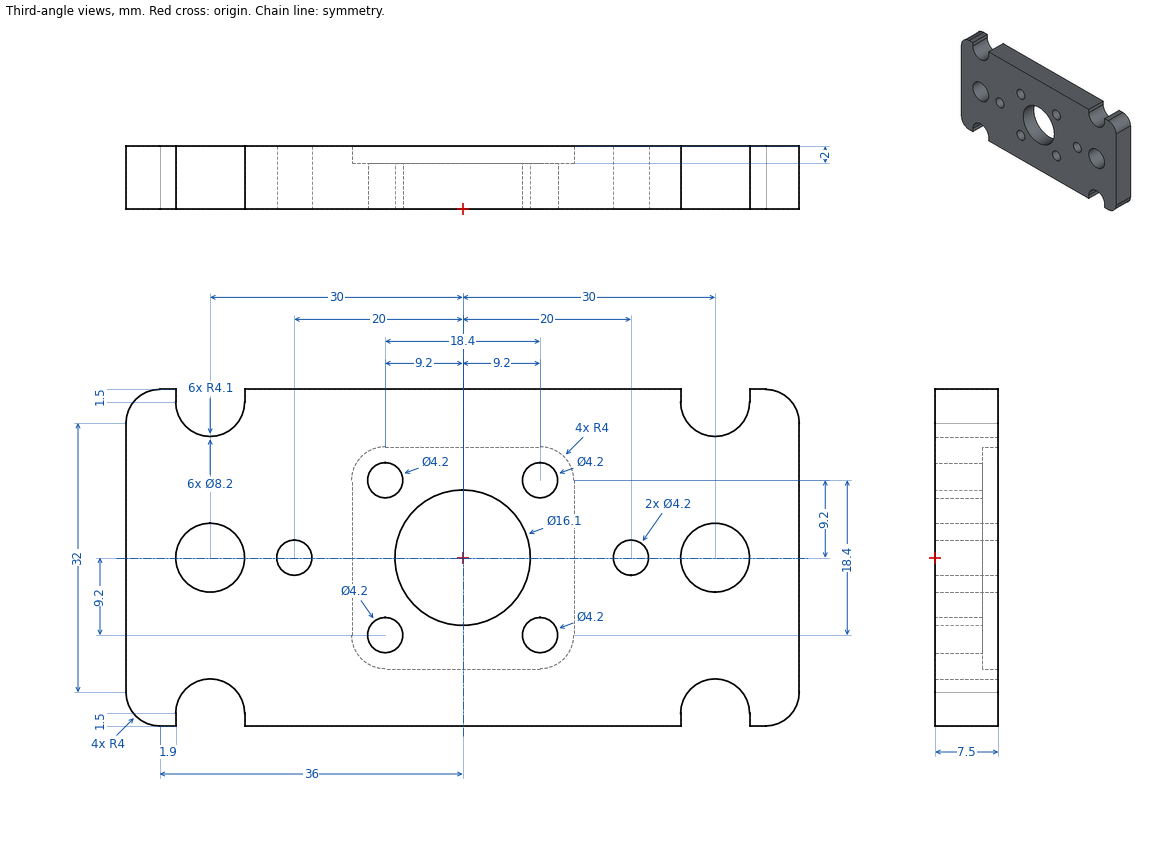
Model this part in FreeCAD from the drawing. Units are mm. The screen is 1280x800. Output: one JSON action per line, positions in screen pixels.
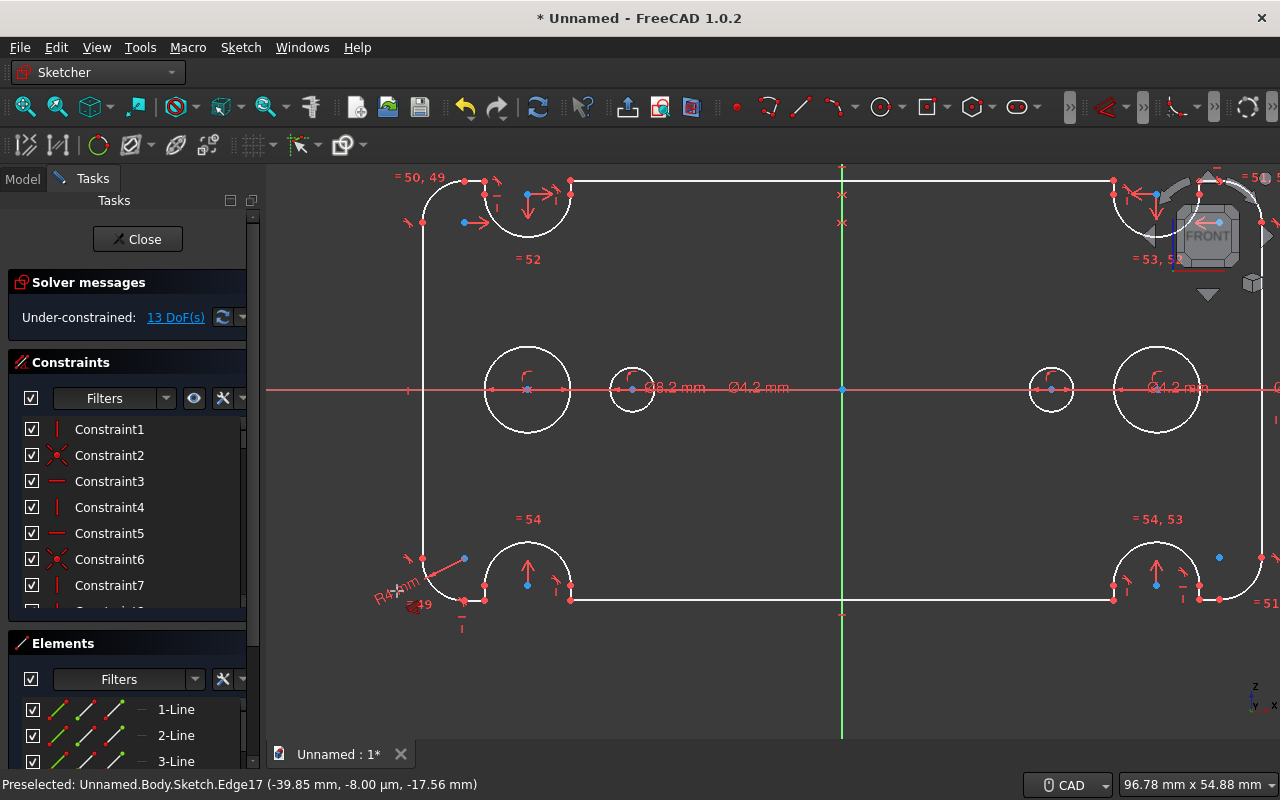
{"action": "left_click", "coordinate": [503, 229]}
{"action": "left_click", "coordinate": [484, 255]}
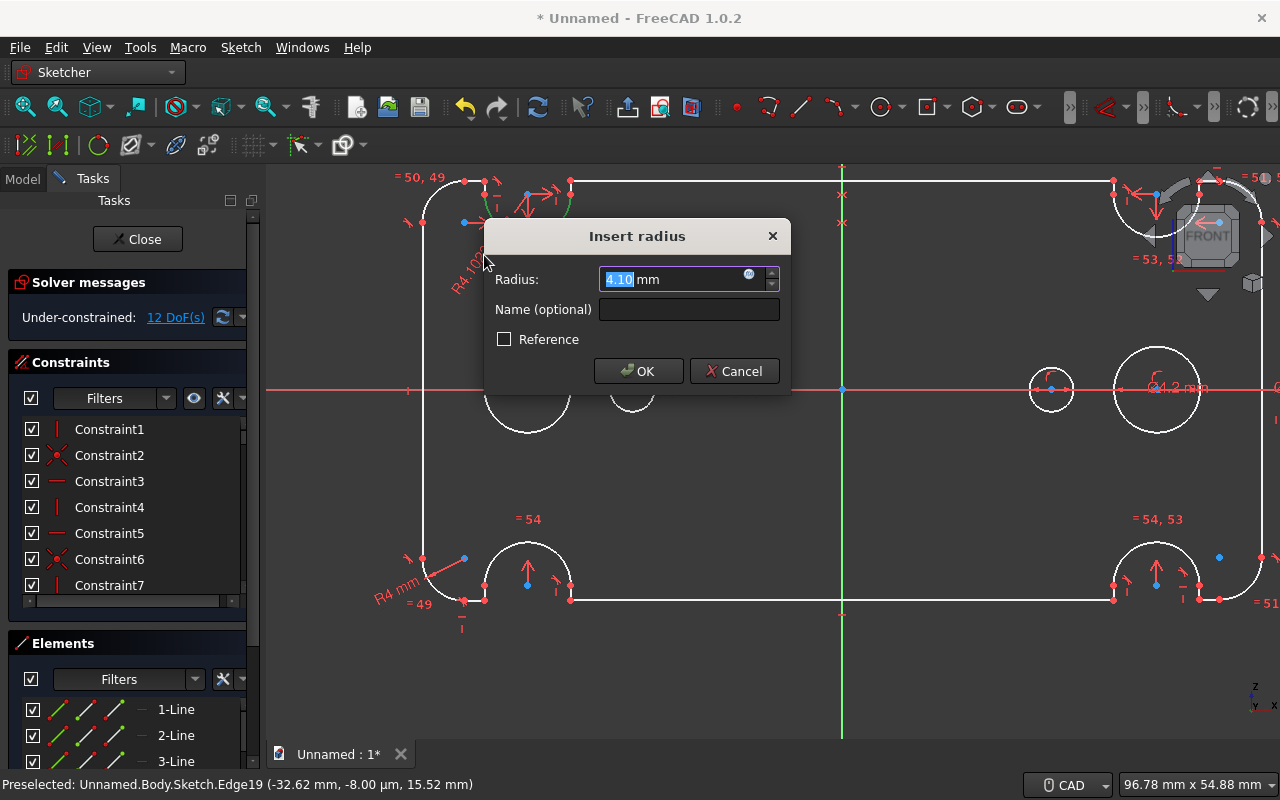
{"action": "type", "text": "4.1"}
{"action": "key", "text": "Return"}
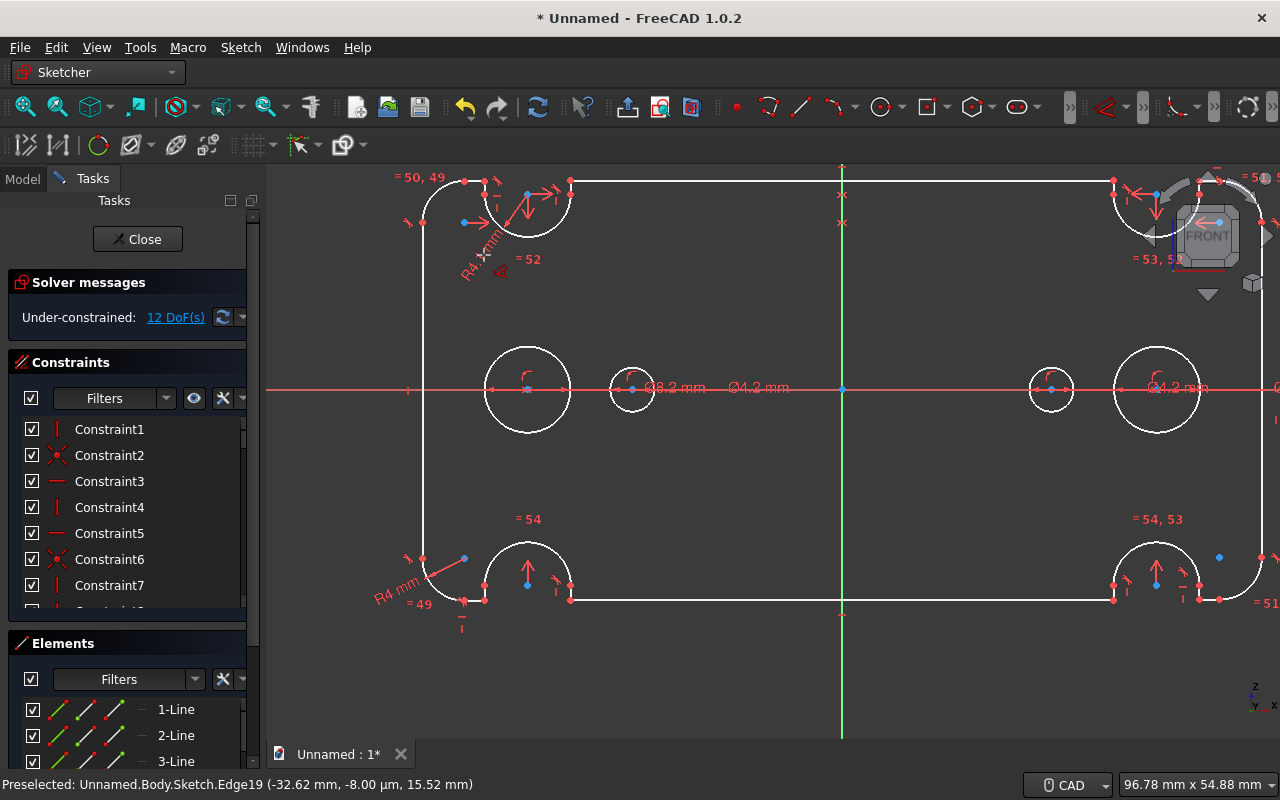
{"action": "left_click", "coordinate": [423, 458]}
{"action": "left_click", "coordinate": [389, 314]}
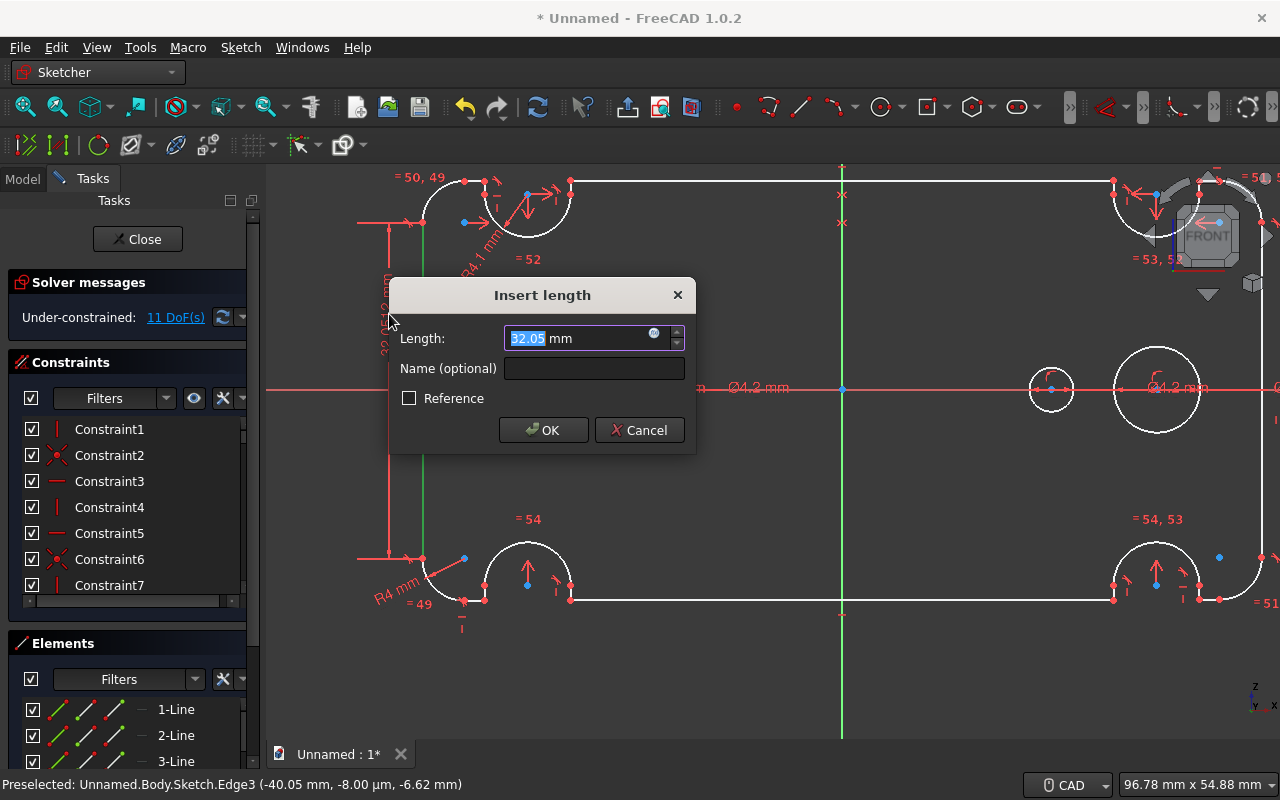
{"action": "type", "text": "32"}
{"action": "key", "text": "Return"}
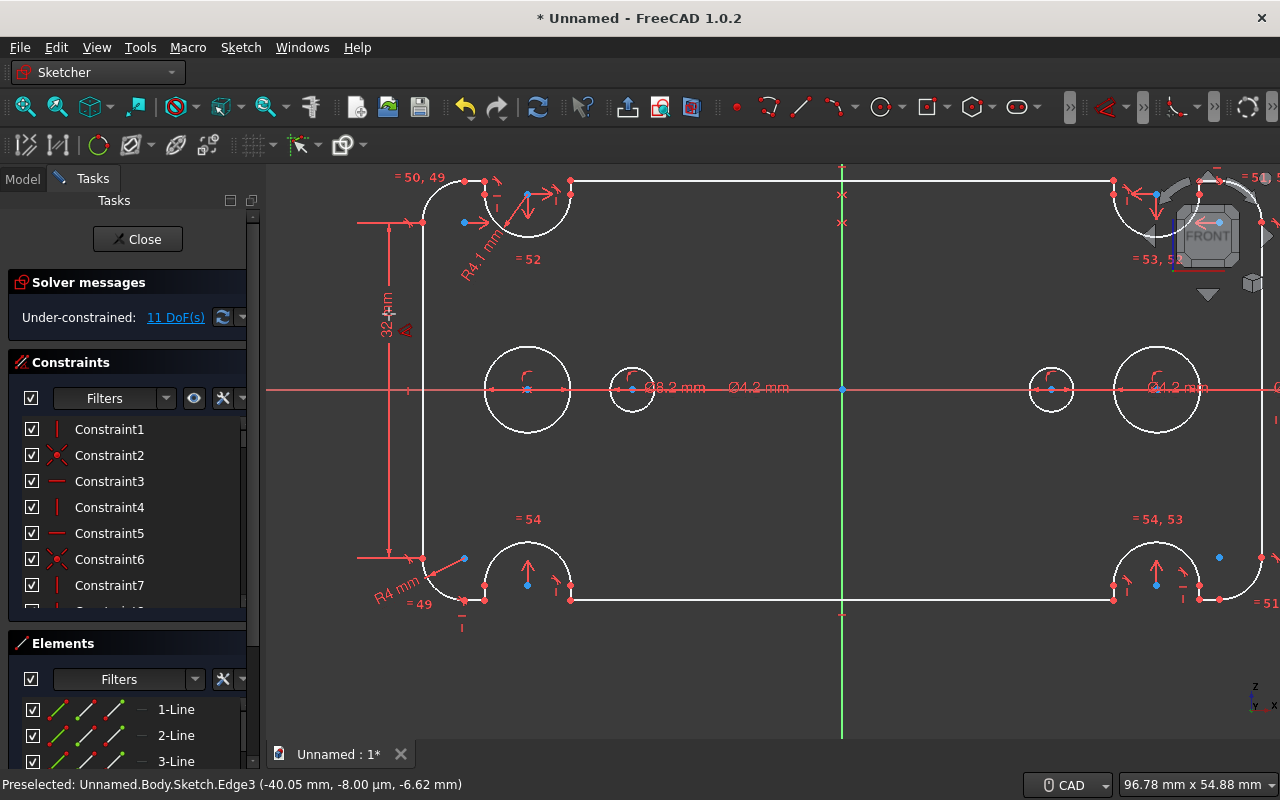
{"action": "scroll", "coordinate": [425, 577], "scroll_direction": "down", "scroll_amount": 2}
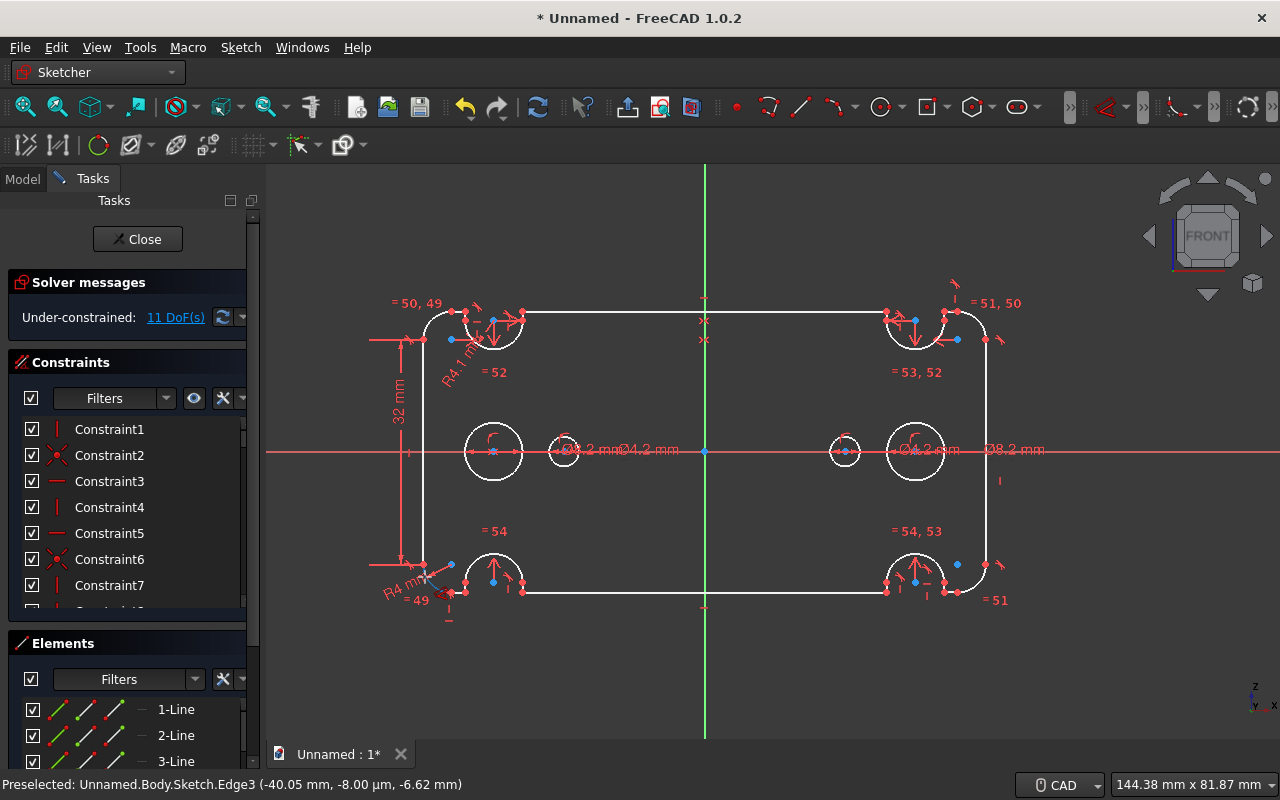
{"action": "left_click", "coordinate": [986, 407]}
{"action": "left_click", "coordinate": [1020, 400]}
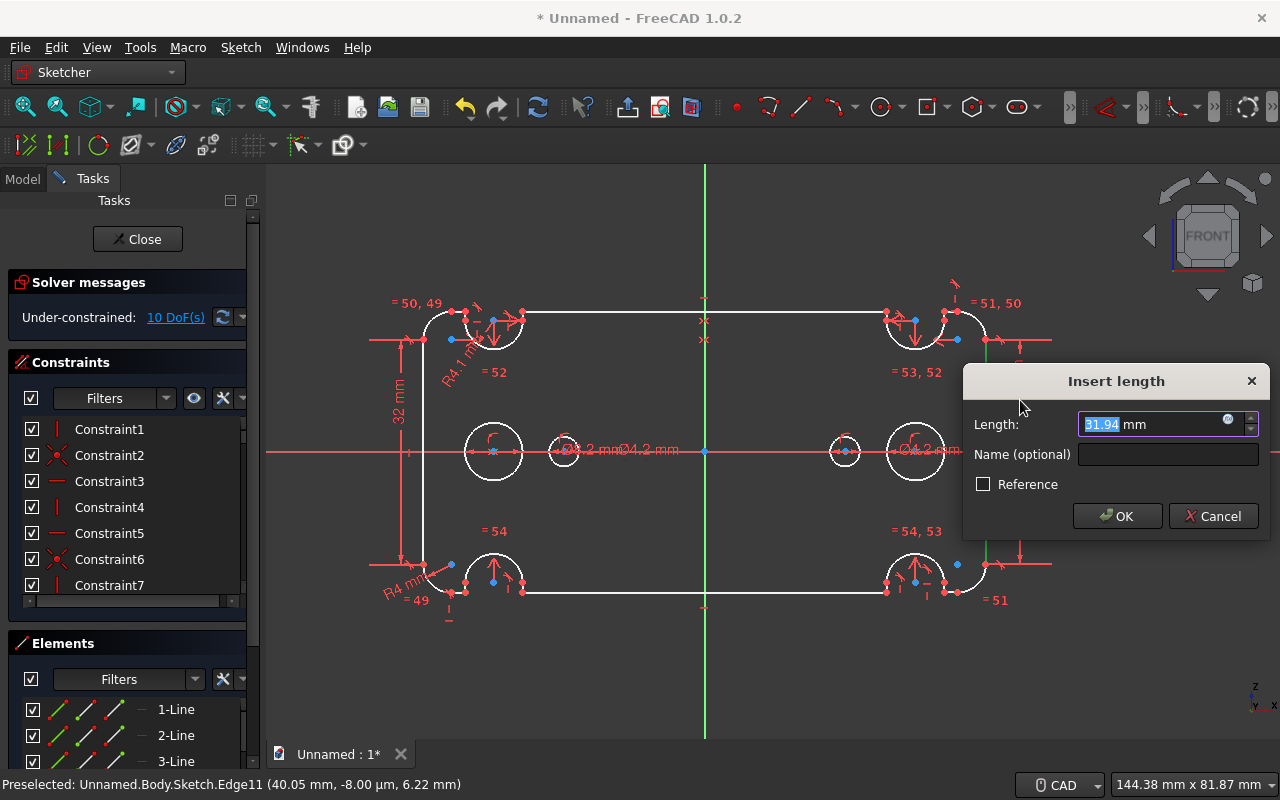
{"action": "type", "text": "32"}
{"action": "key", "text": "Return"}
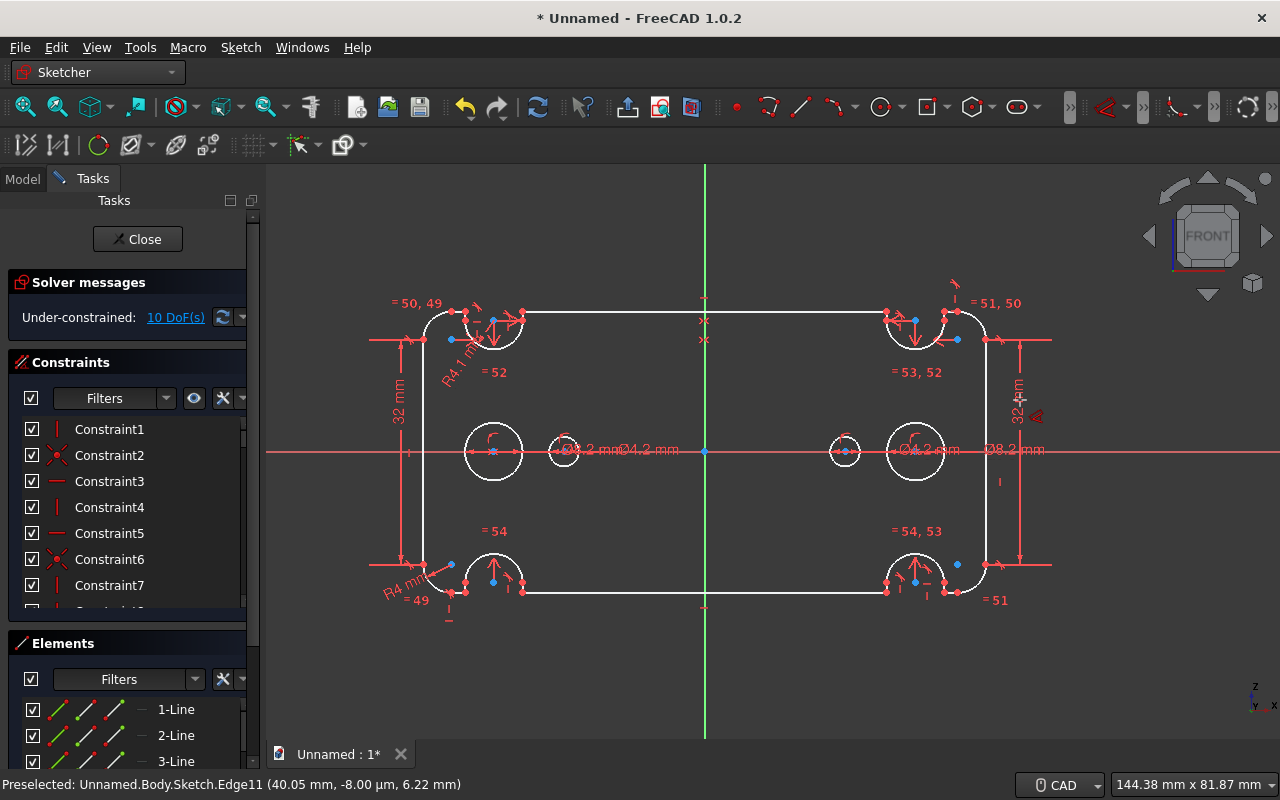
{"action": "left_click", "coordinate": [916, 452]}
{"action": "left_click", "coordinate": [810, 486]}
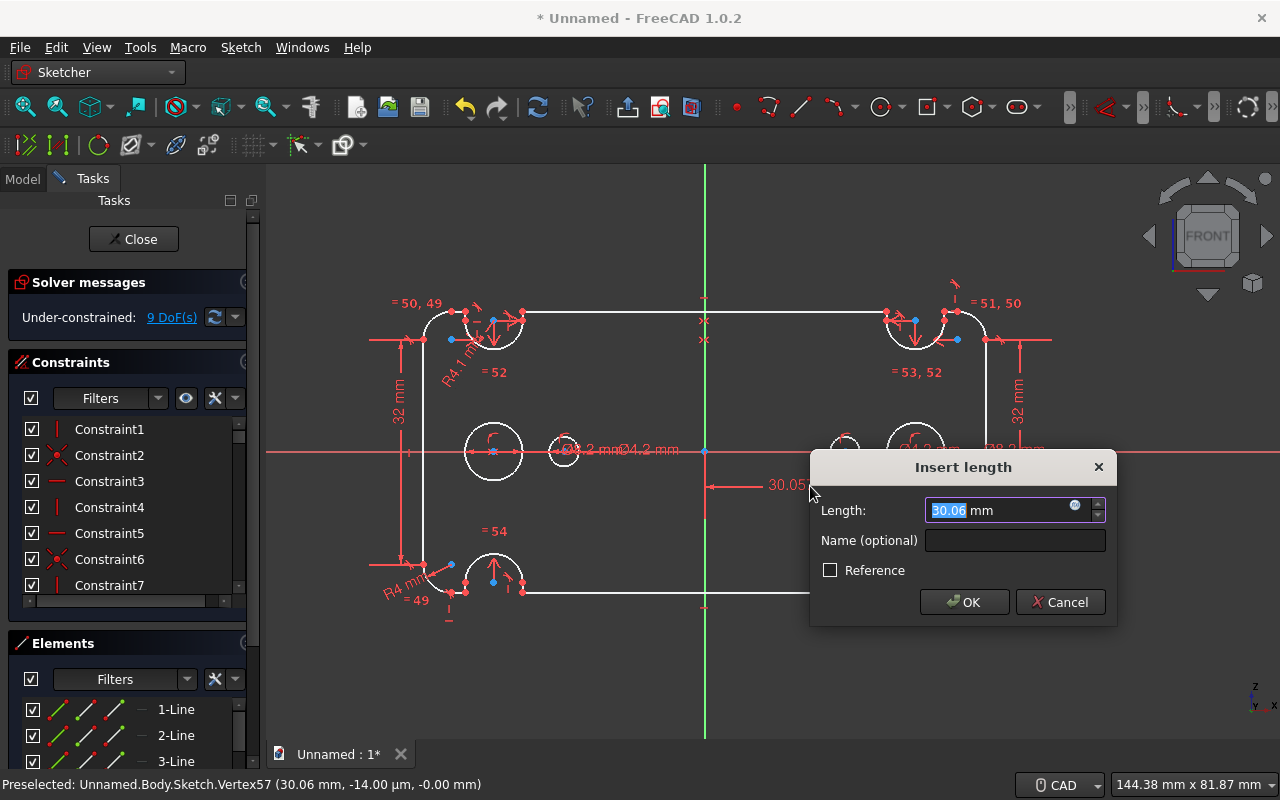
{"action": "type", "text": "30"}
{"action": "key", "text": "Return"}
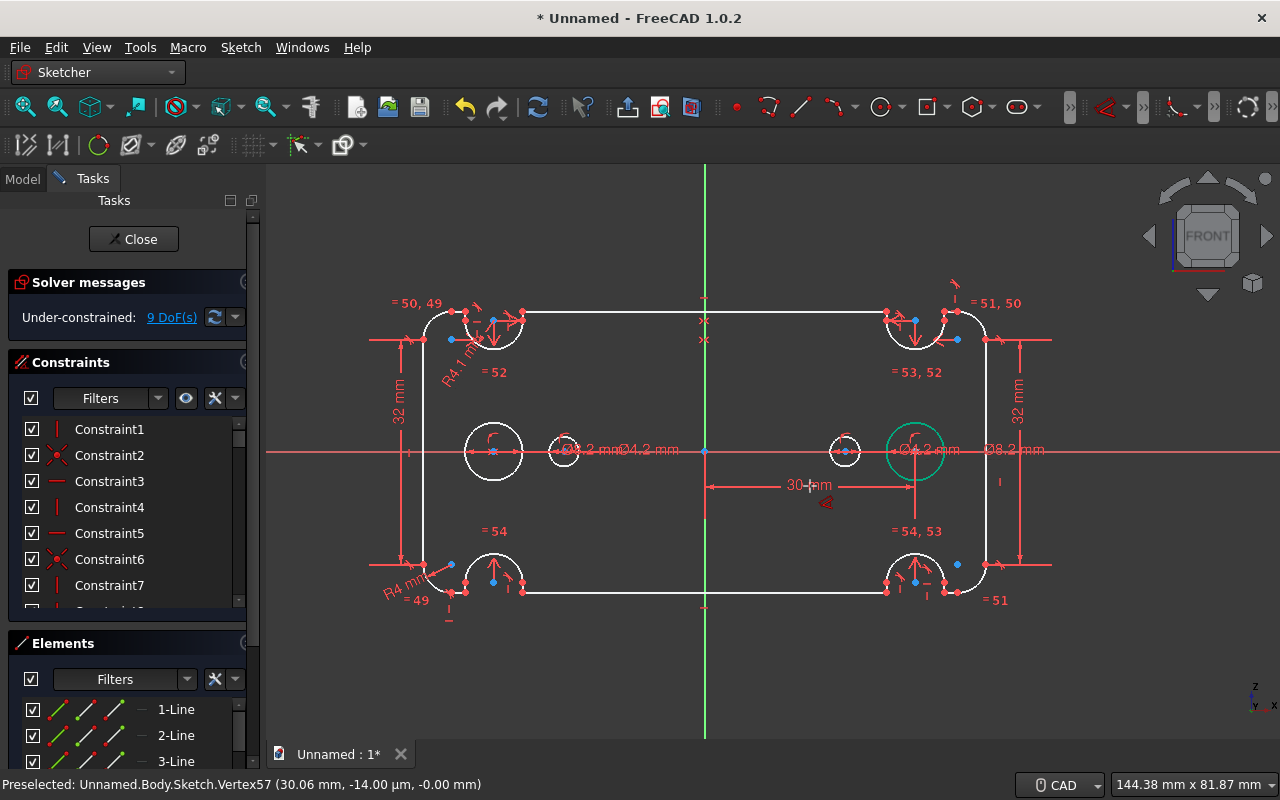
{"action": "left_click", "coordinate": [845, 452]}
{"action": "left_click", "coordinate": [726, 486]}